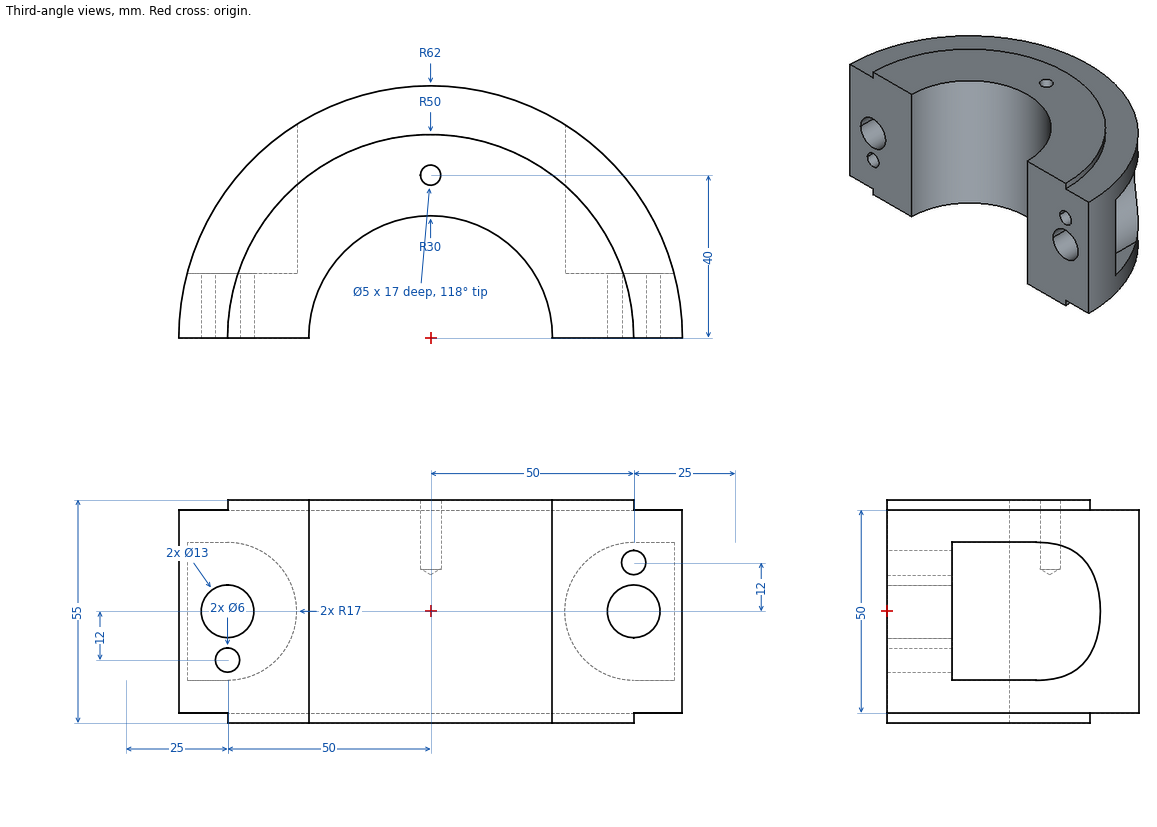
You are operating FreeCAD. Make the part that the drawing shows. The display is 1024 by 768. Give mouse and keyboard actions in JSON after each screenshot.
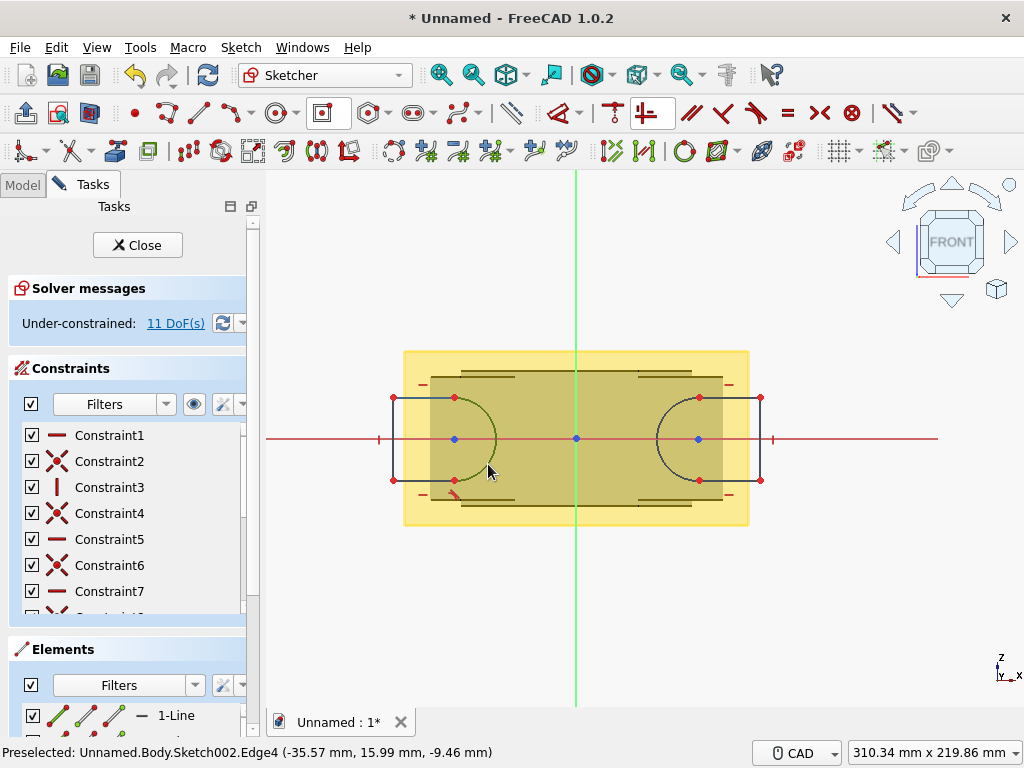
{"action": "left_click", "coordinate": [756, 114]}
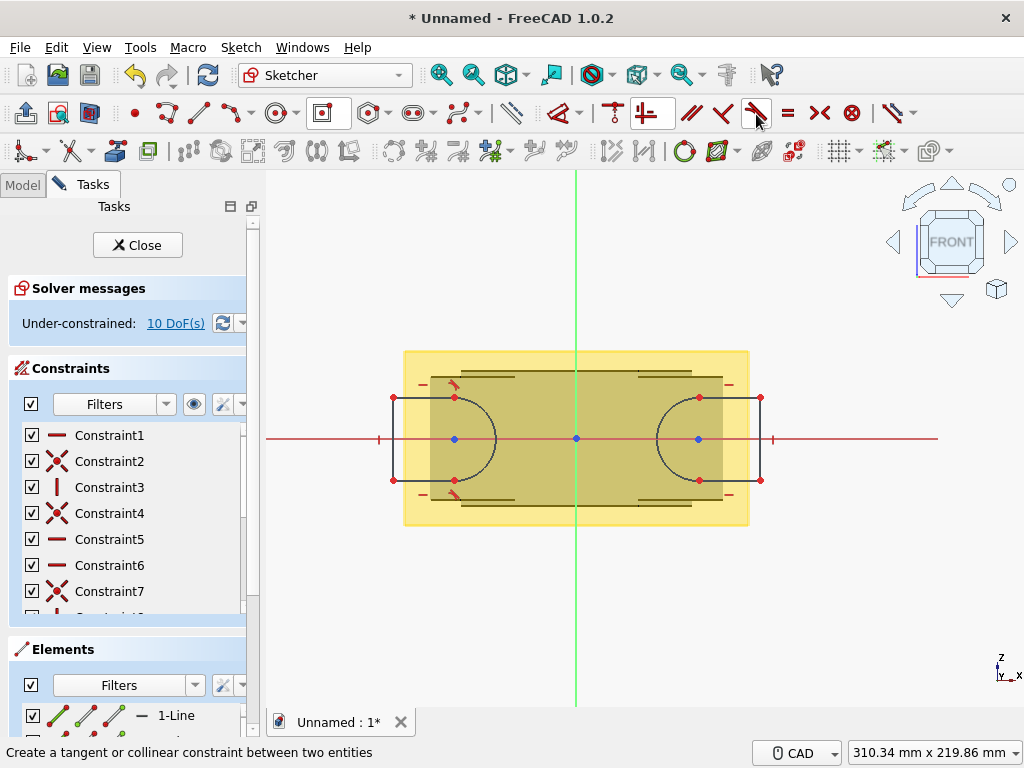
{"action": "left_click", "coordinate": [717, 398]}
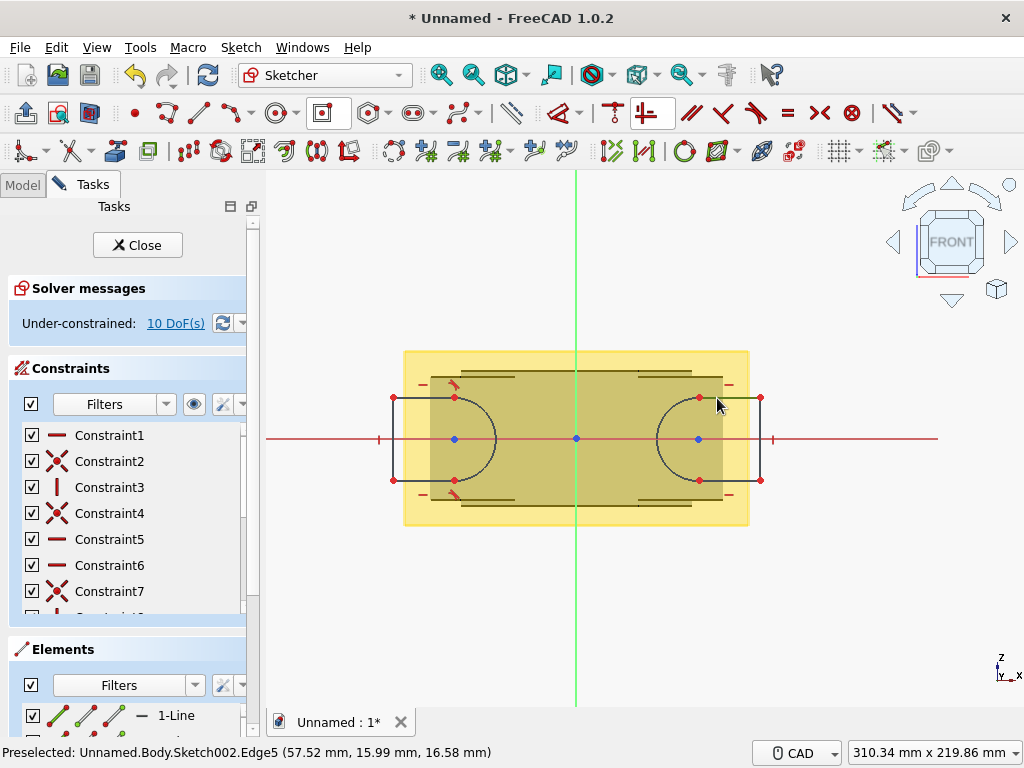
{"action": "left_click", "coordinate": [665, 415]}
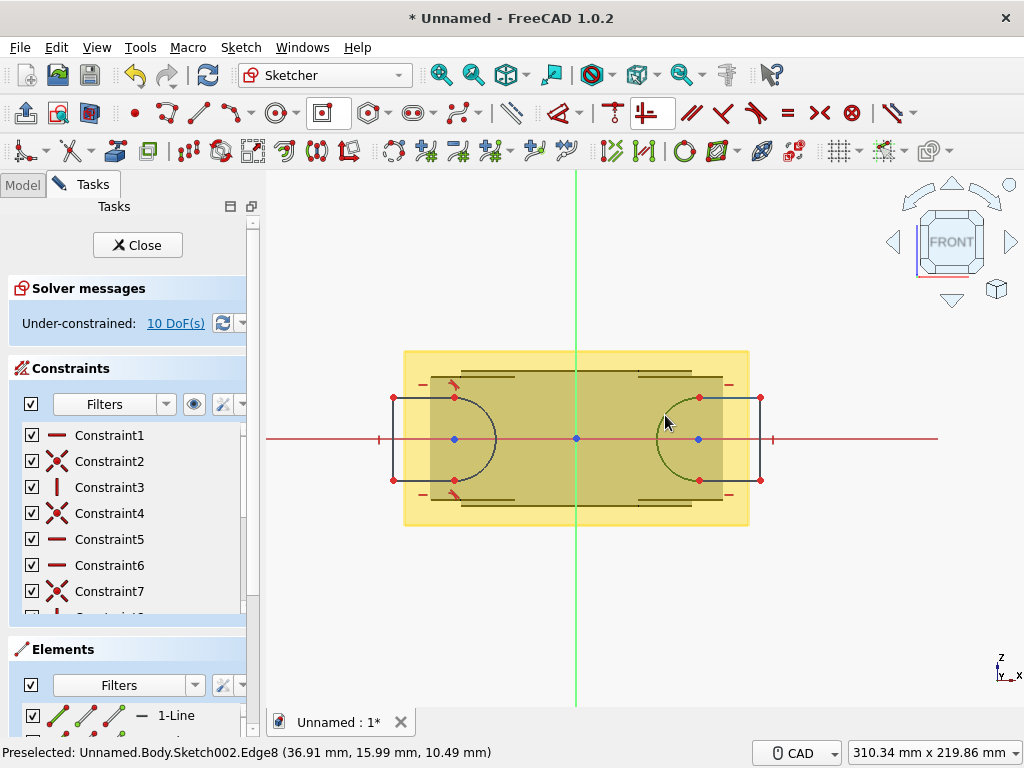
{"action": "left_click", "coordinate": [756, 114]}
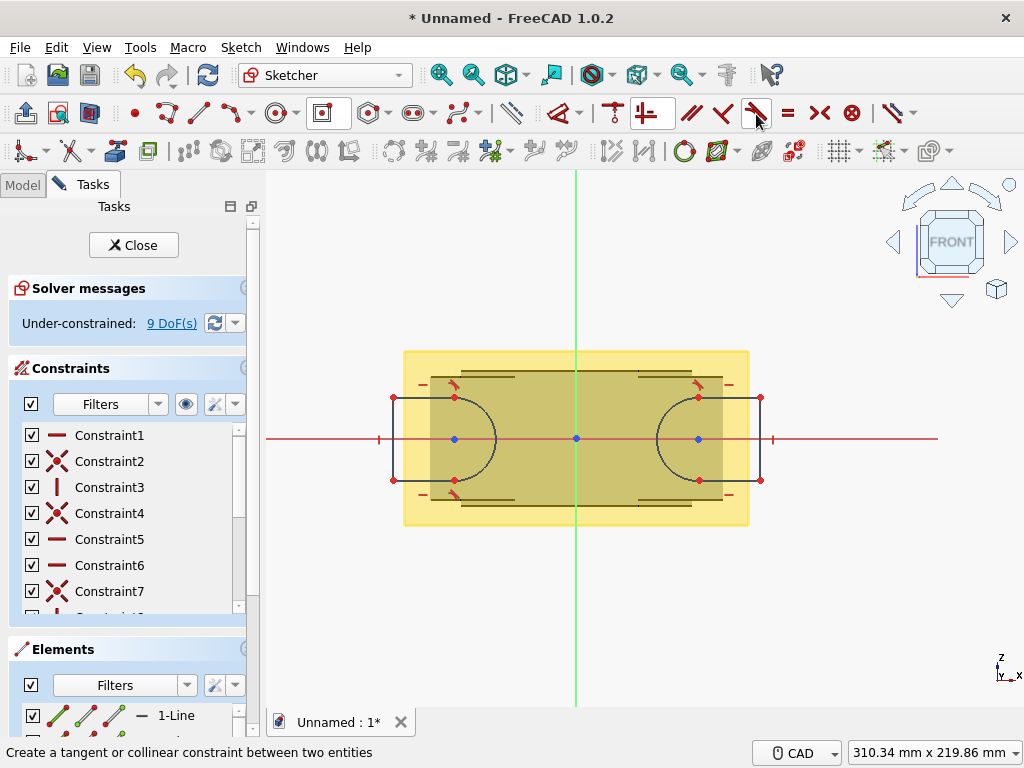
{"action": "left_click", "coordinate": [742, 481]}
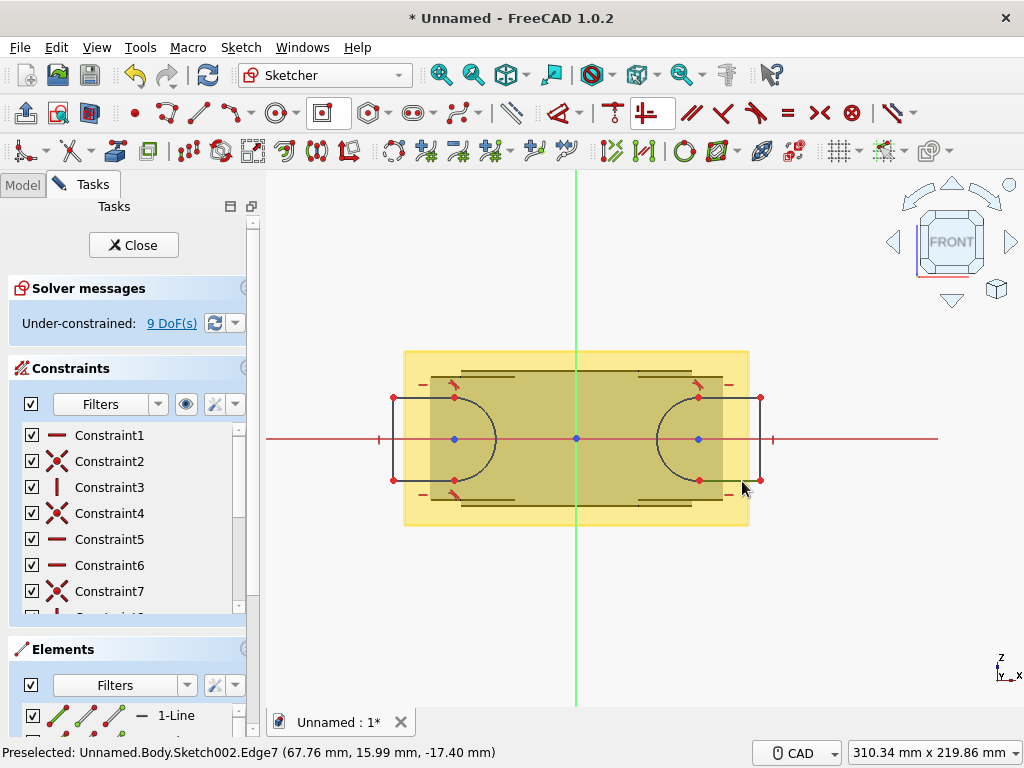
{"action": "left_click", "coordinate": [665, 415]}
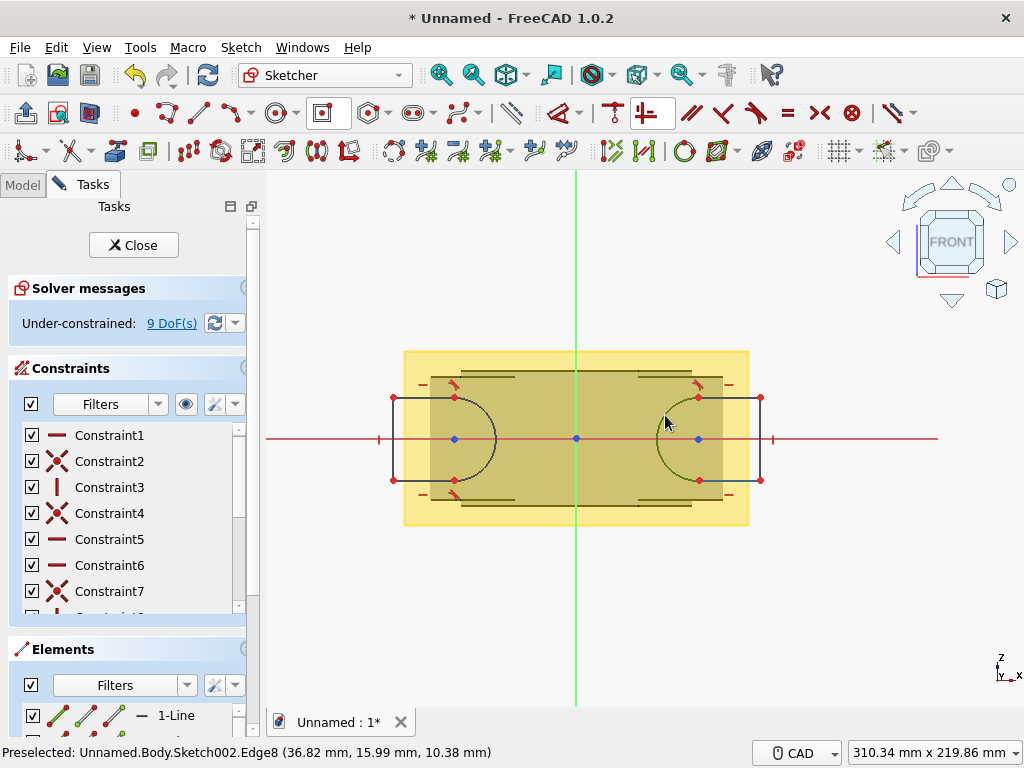
{"action": "left_click", "coordinate": [756, 114]}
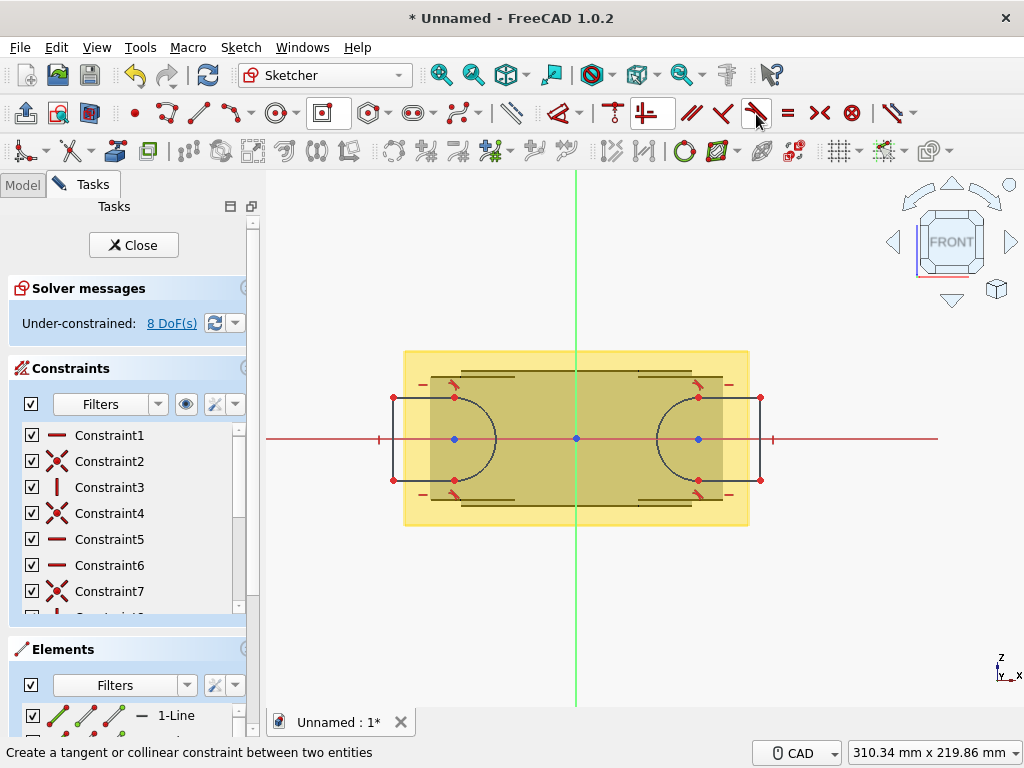
{"action": "left_click", "coordinate": [488, 464]}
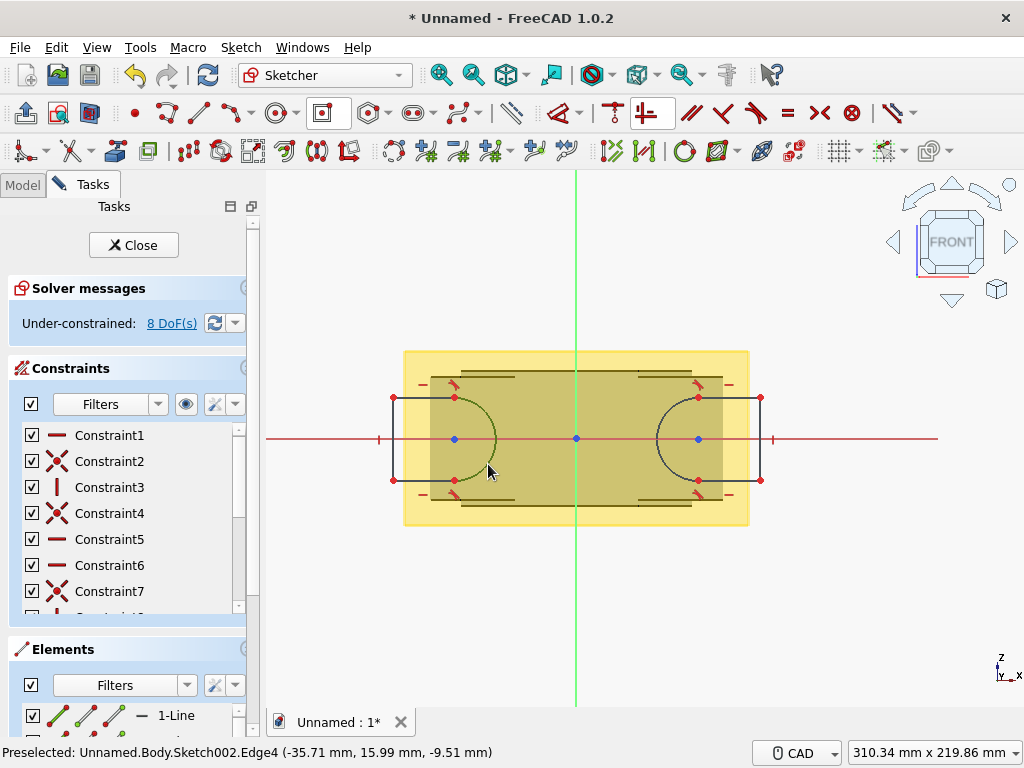
{"action": "left_click", "coordinate": [665, 415]}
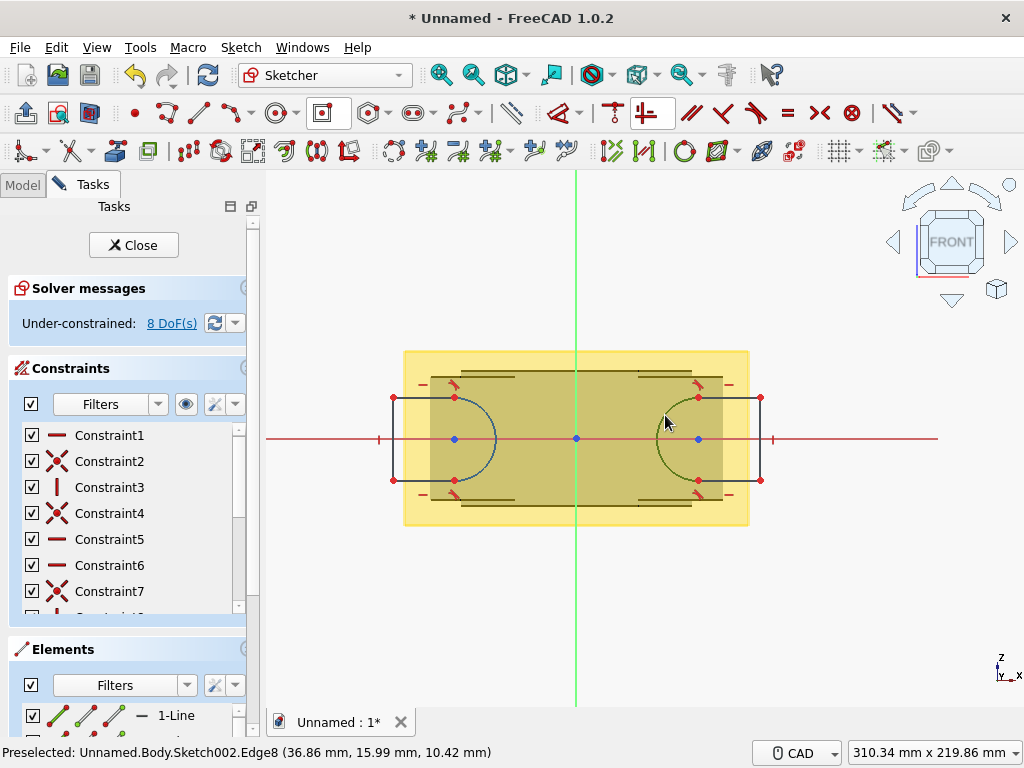
{"action": "left_click", "coordinate": [788, 114]}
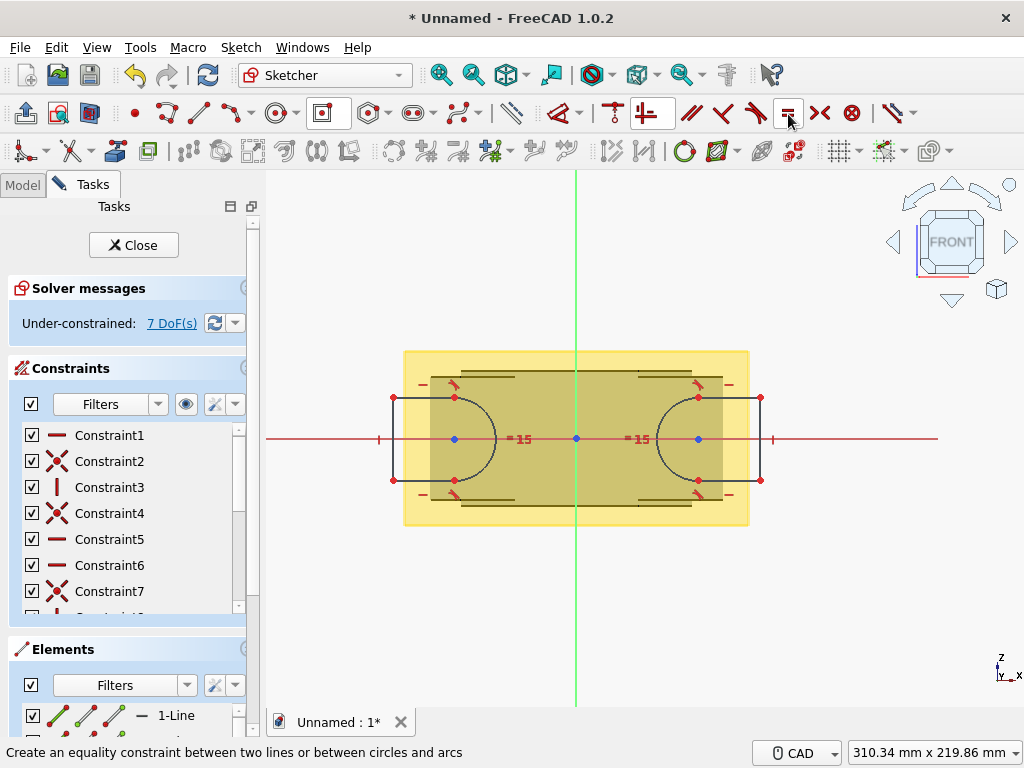
{"action": "left_click", "coordinate": [454, 439]}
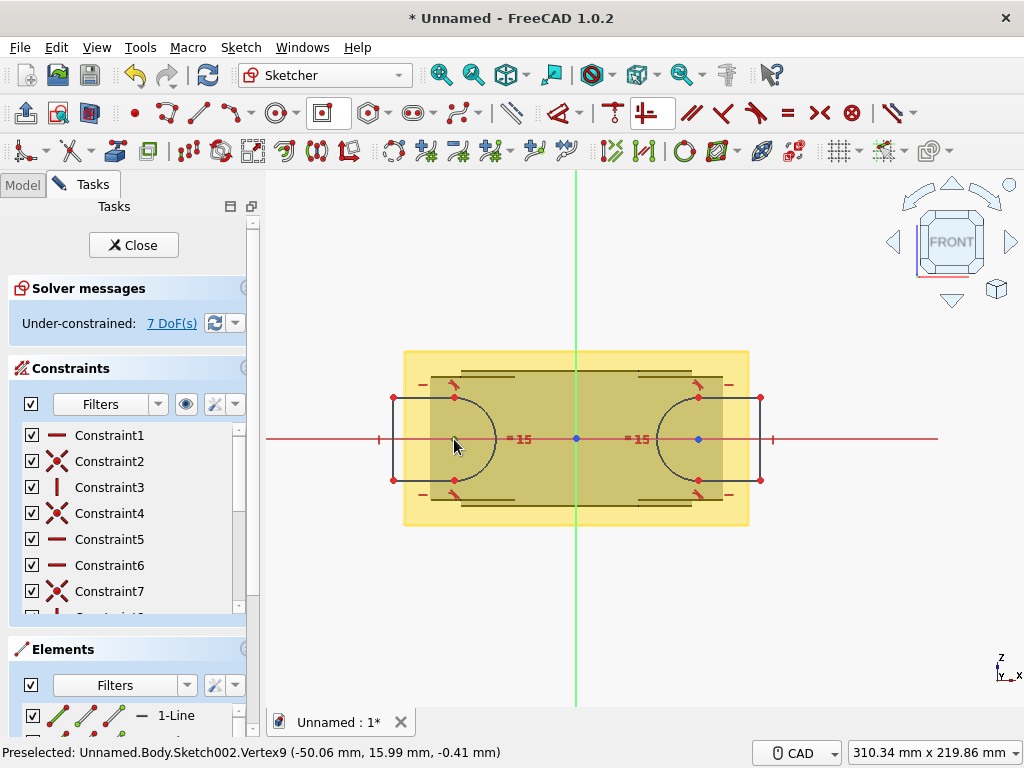
{"action": "left_click", "coordinate": [334, 439]}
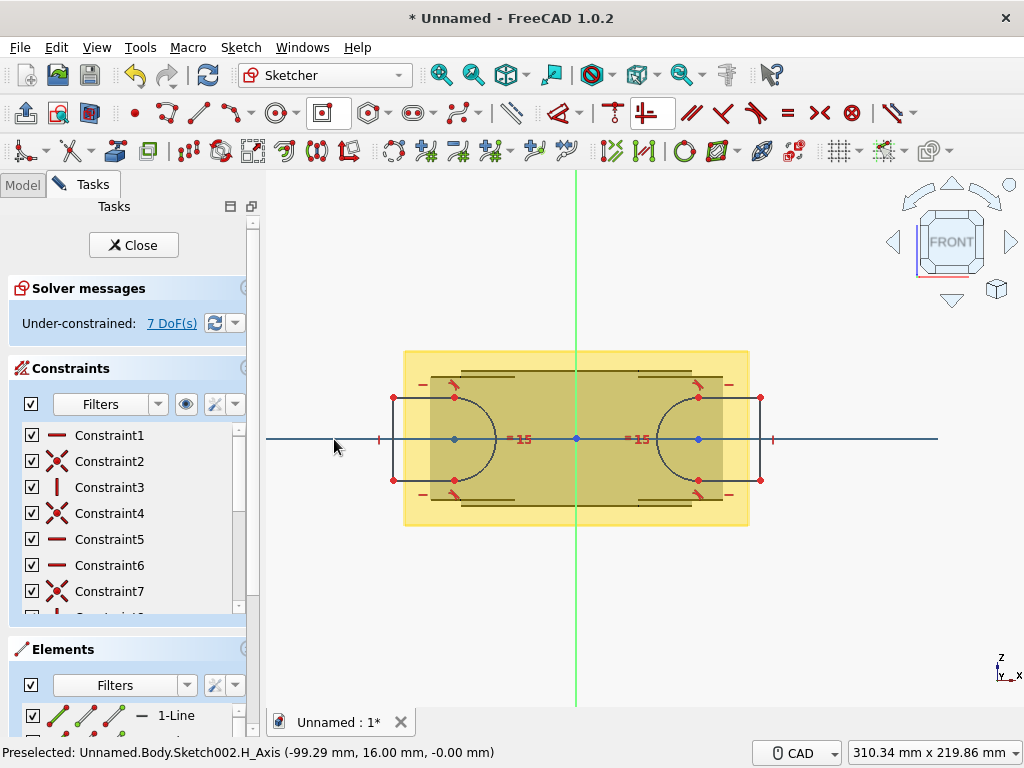
{"action": "left_click", "coordinate": [614, 114]}